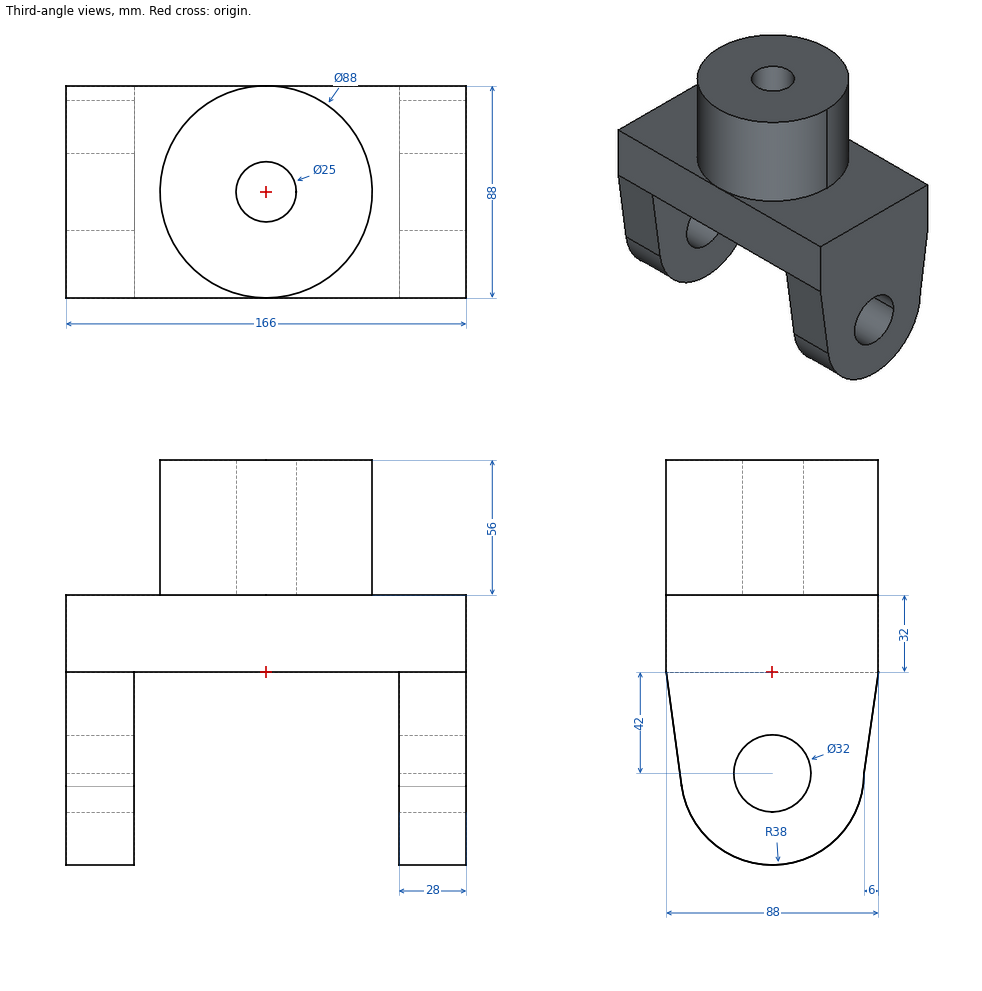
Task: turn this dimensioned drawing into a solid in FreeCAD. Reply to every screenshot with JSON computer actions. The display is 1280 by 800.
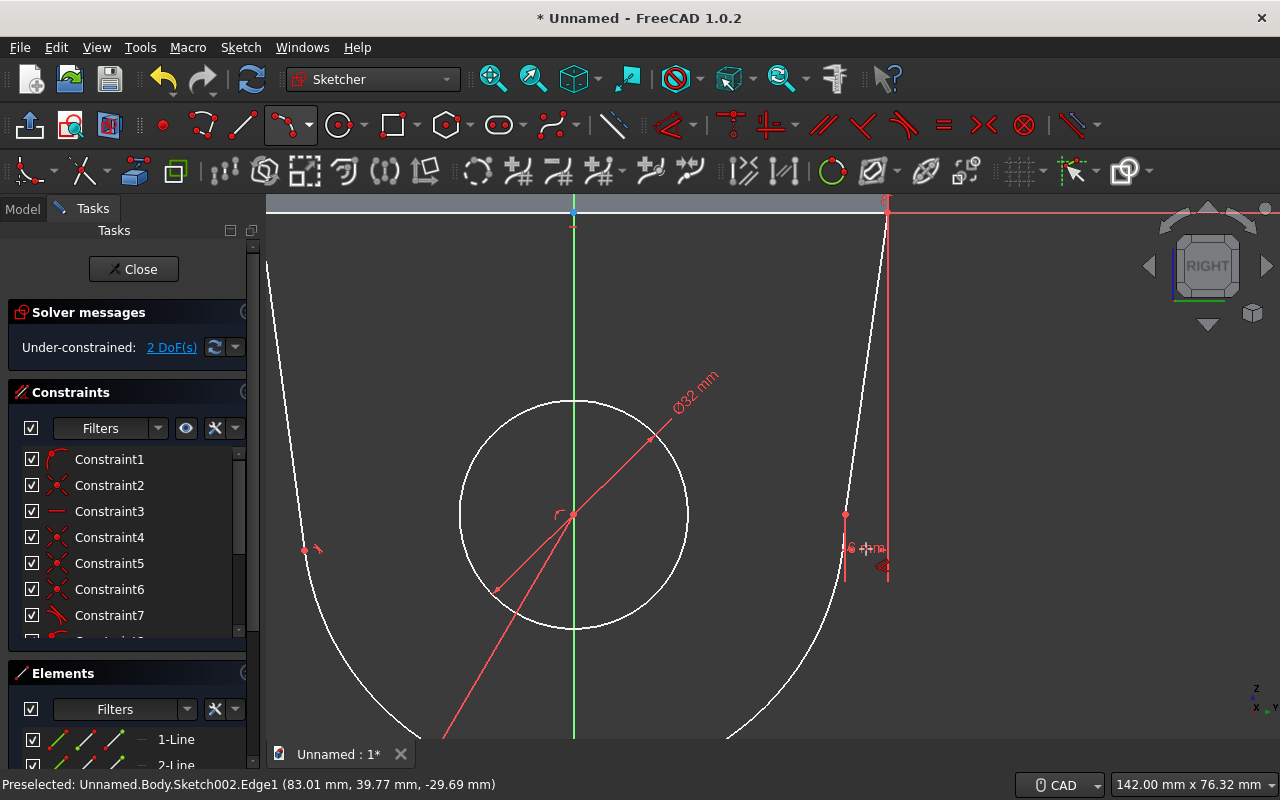
{"action": "left_click", "coordinate": [574, 515]}
{"action": "left_click", "coordinate": [608, 368]}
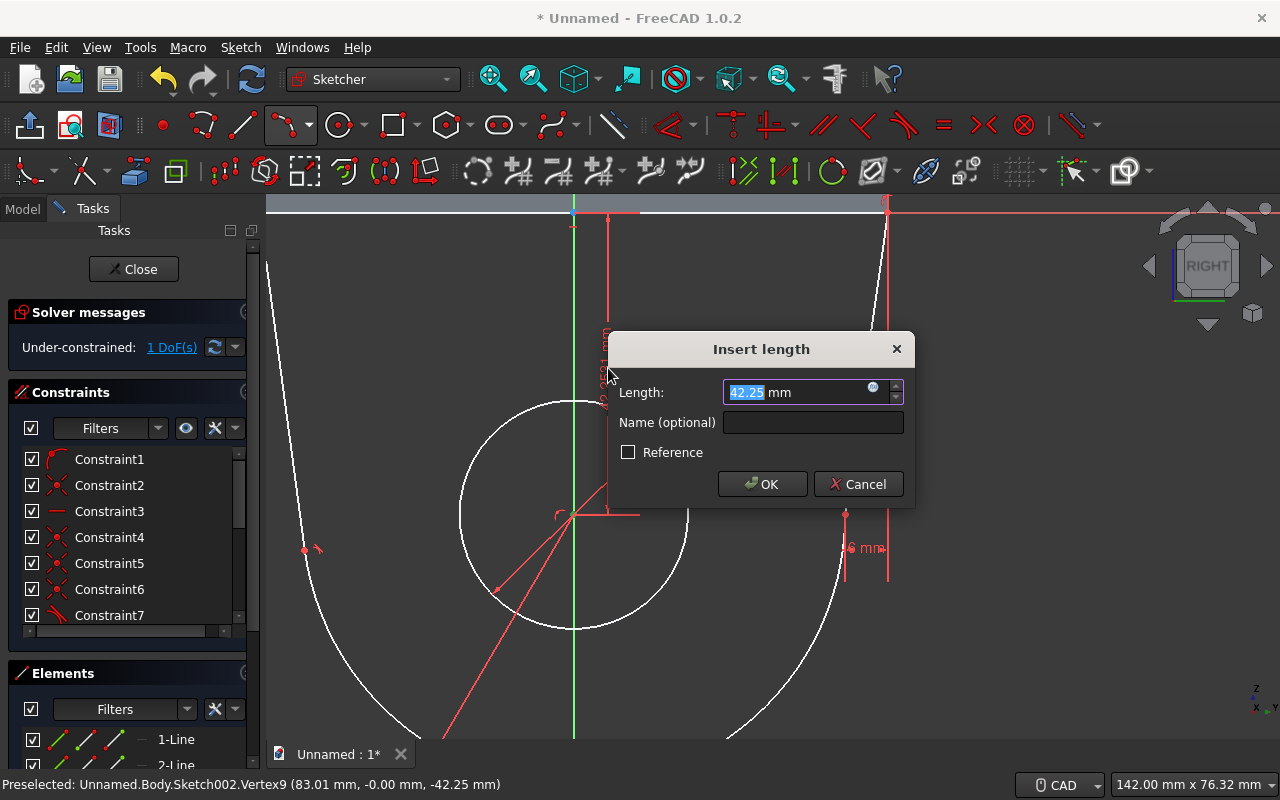
{"action": "type", "text": "42"}
{"action": "key", "text": "Return"}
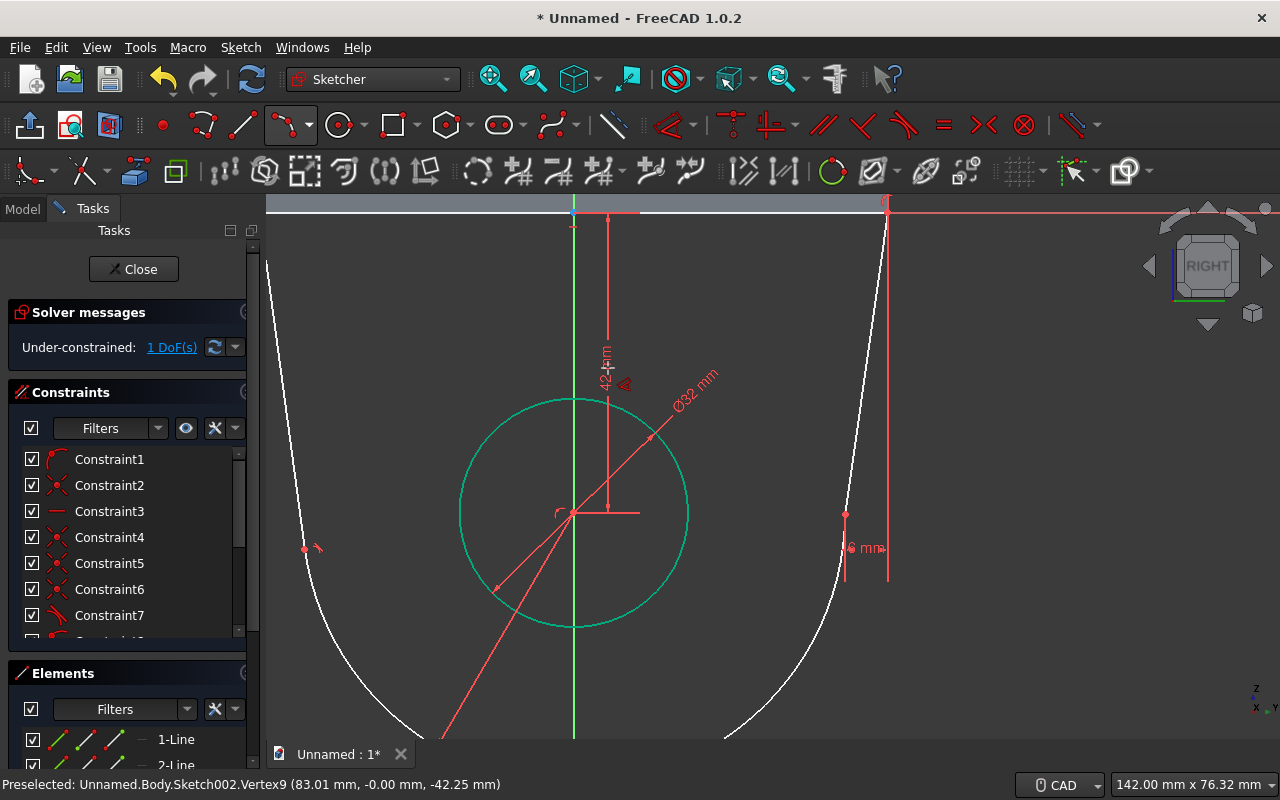
{"action": "left_click", "coordinate": [845, 515]}
{"action": "left_click", "coordinate": [879, 368]}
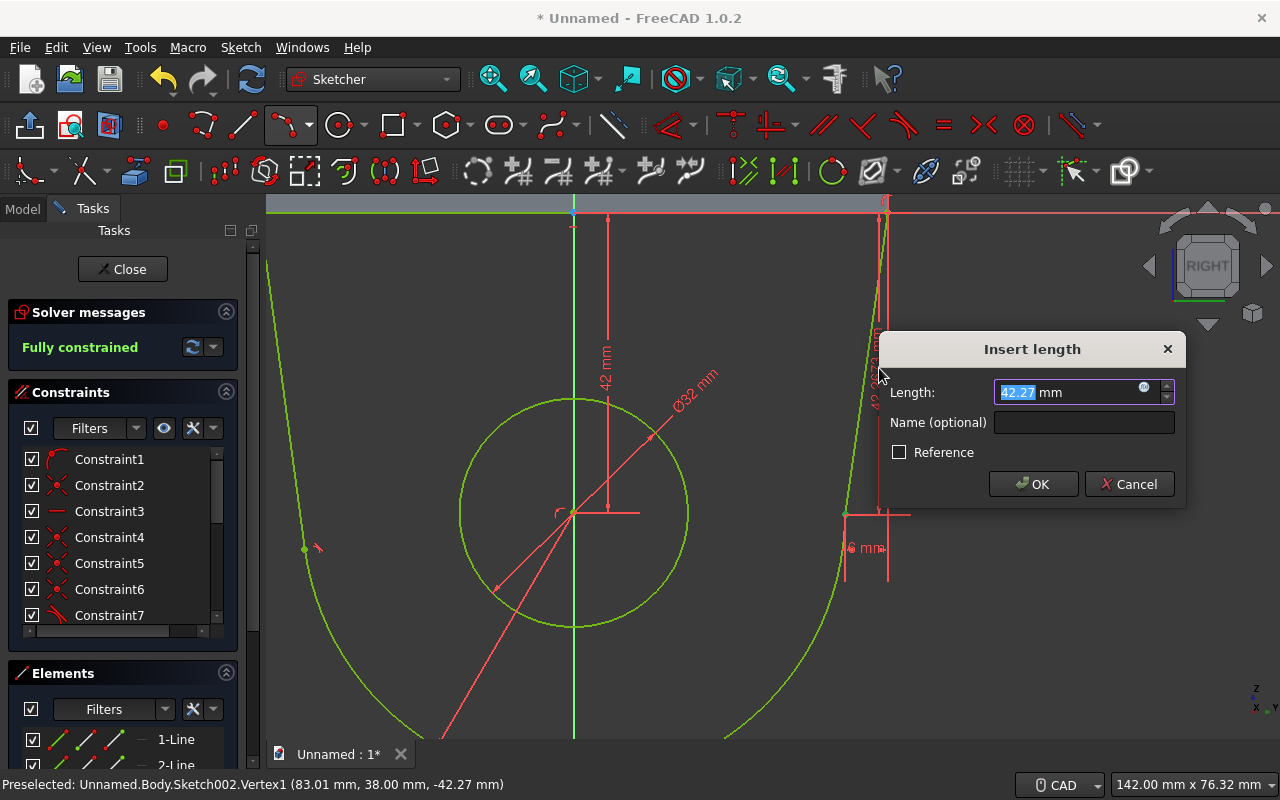
{"action": "type", "text": "42"}
{"action": "key", "text": "Return"}
{"action": "key", "text": "Escape"}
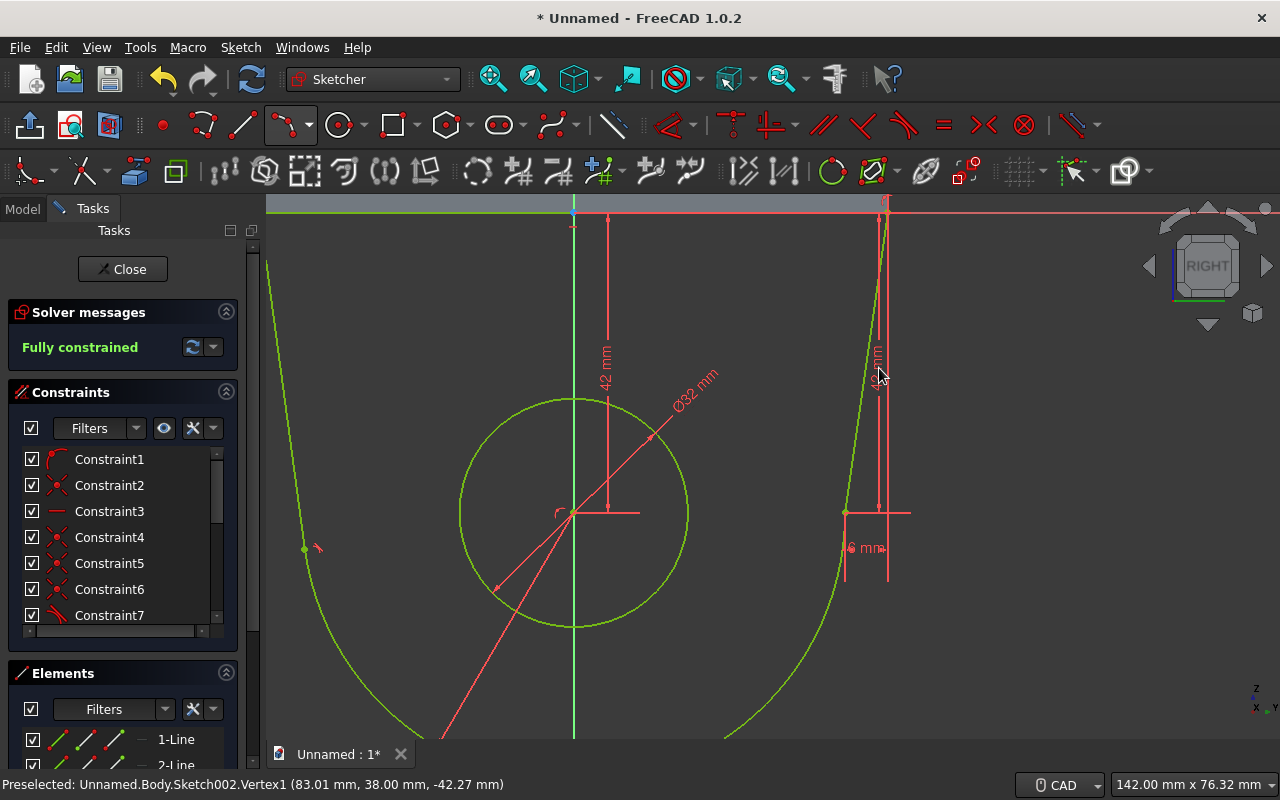
{"action": "left_click", "coordinate": [123, 269]}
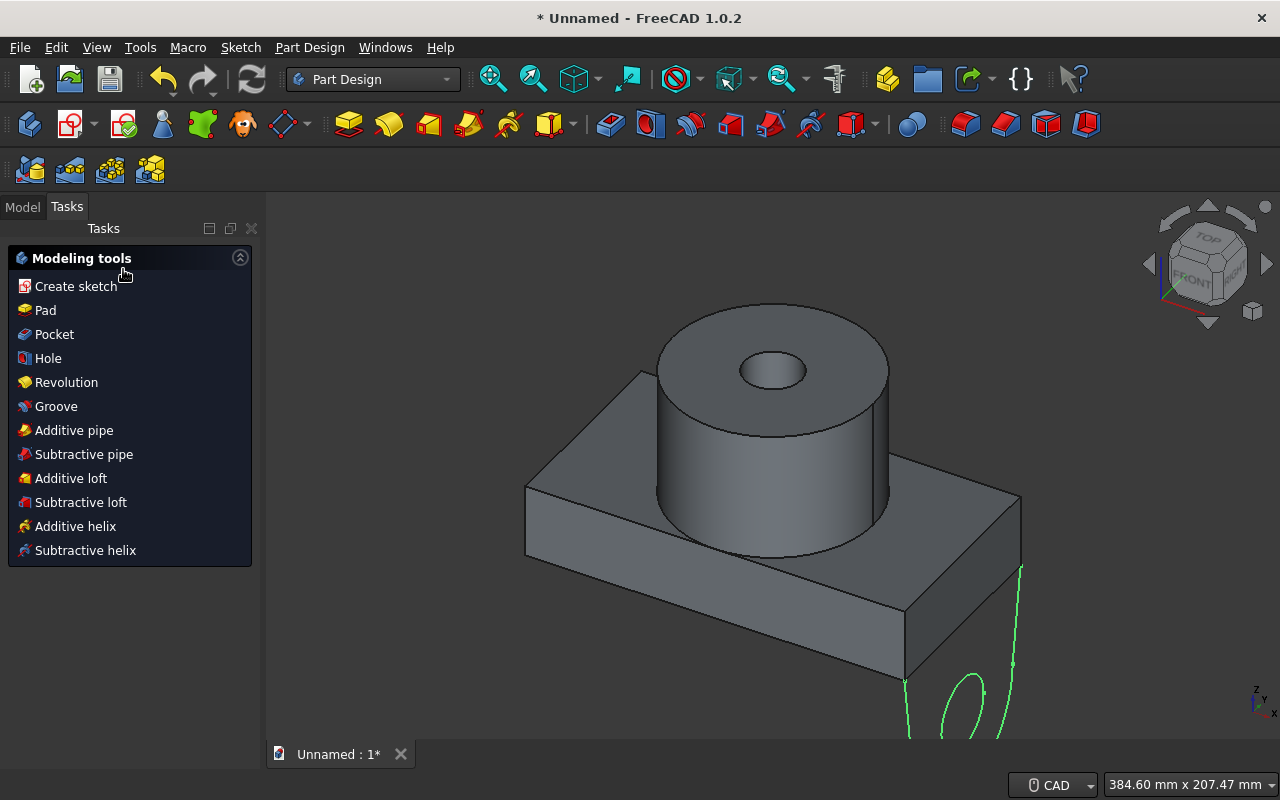
{"action": "left_click", "coordinate": [350, 124]}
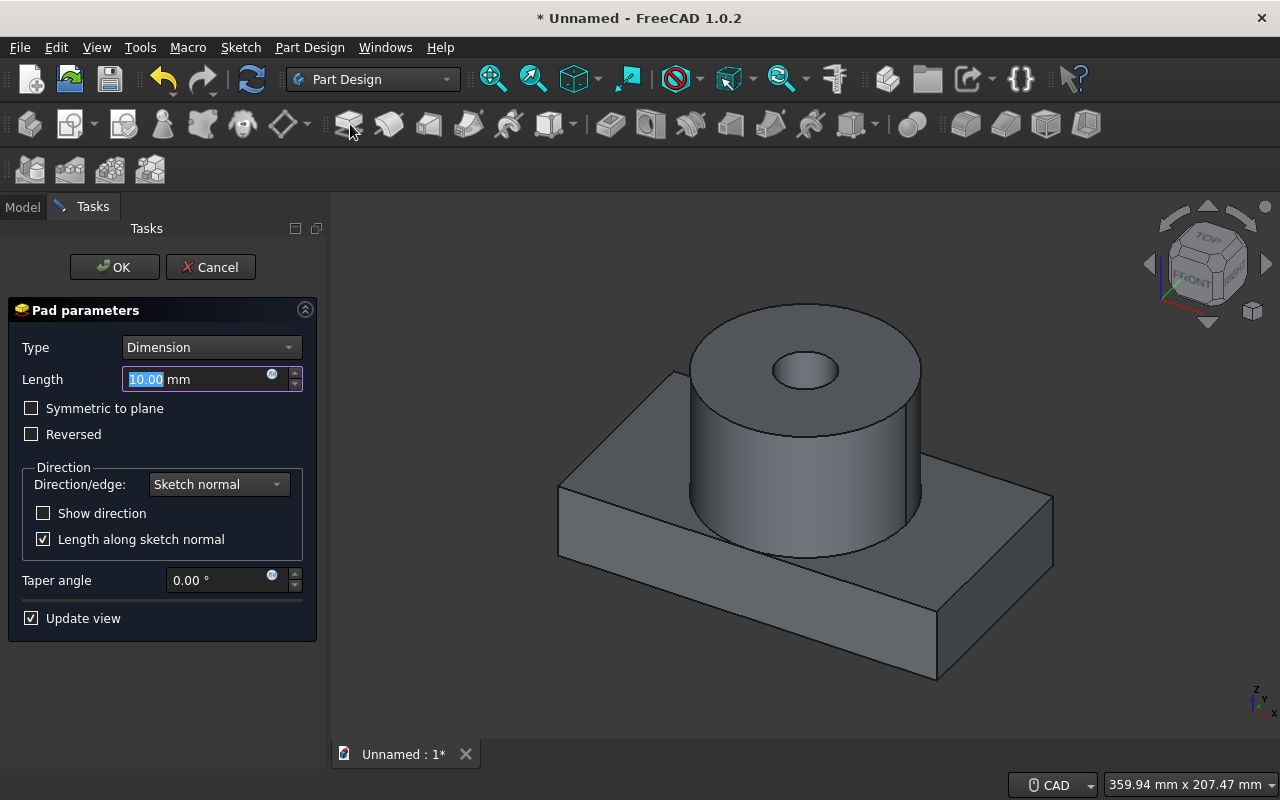
{"action": "type", "text": "28"}
{"action": "key", "text": "Tab"}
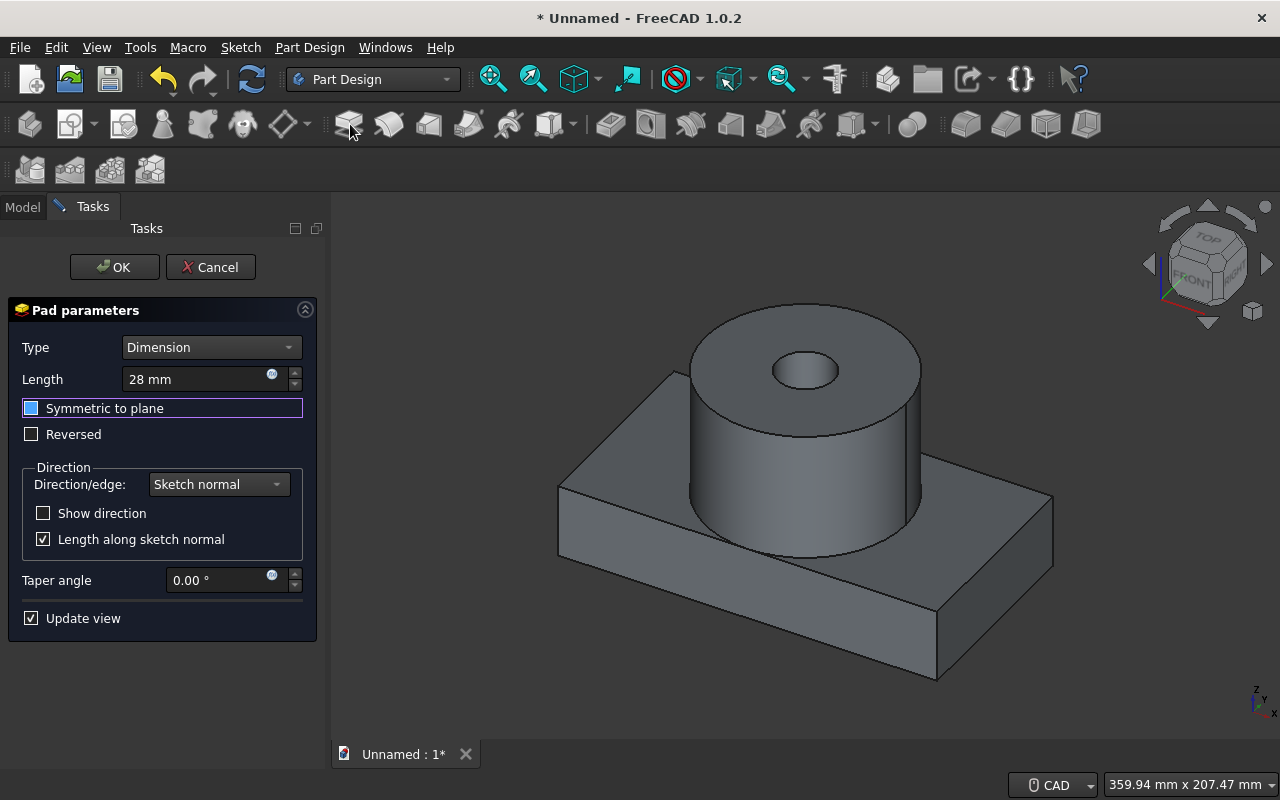
{"action": "left_click", "coordinate": [30, 434]}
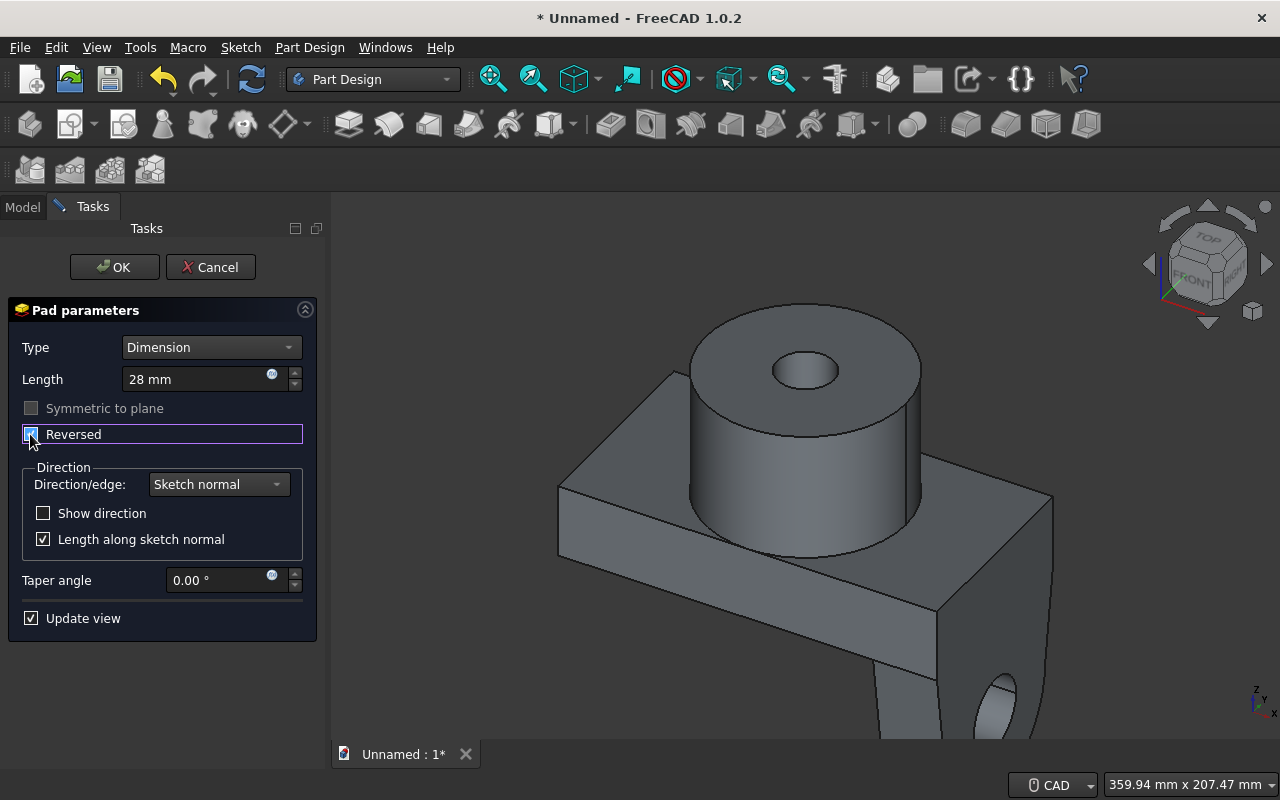
{"action": "left_click", "coordinate": [115, 267]}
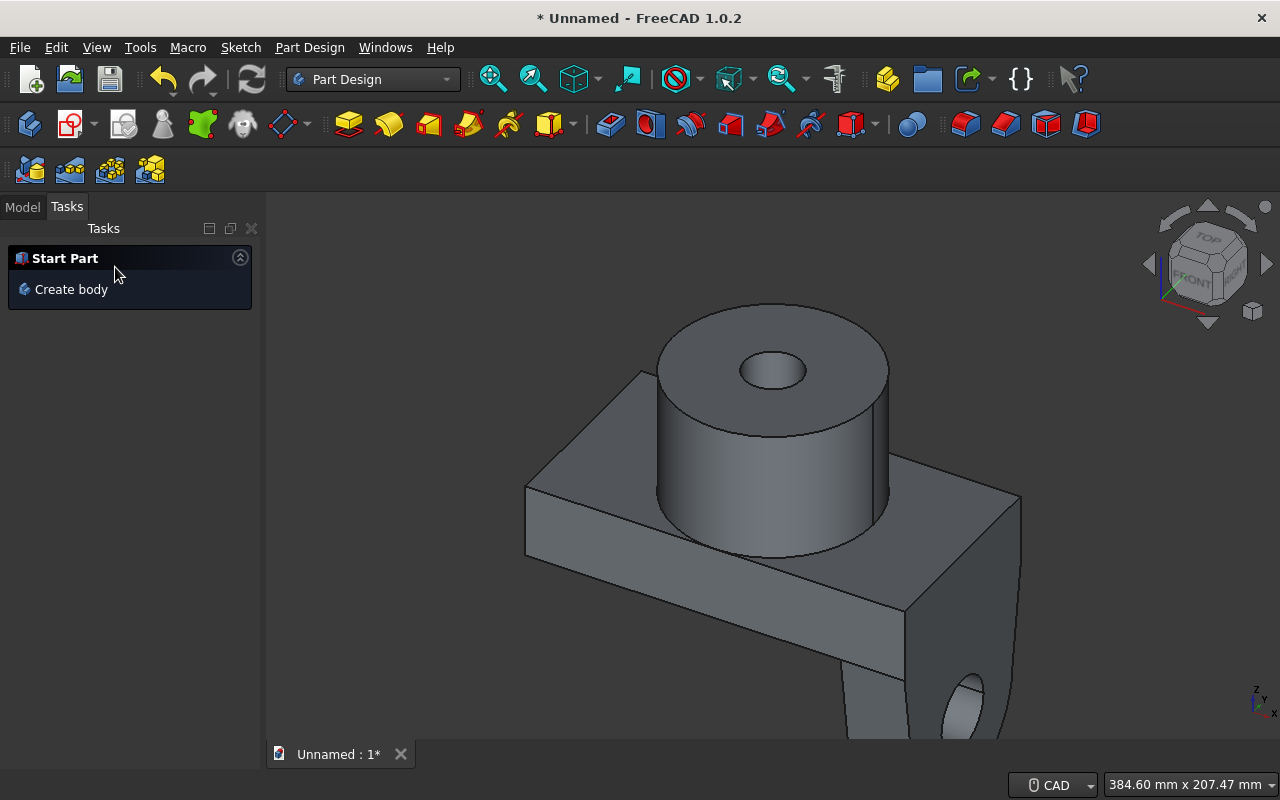
{"action": "left_click", "coordinate": [494, 80]}